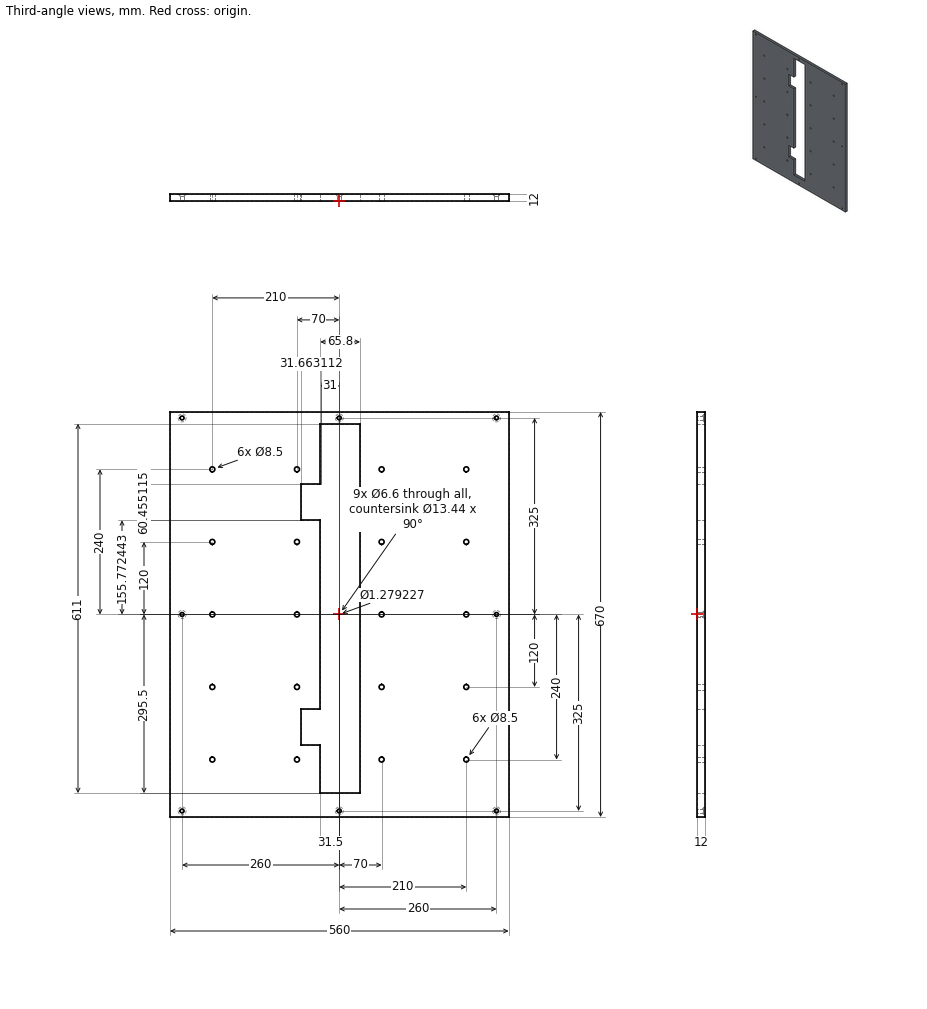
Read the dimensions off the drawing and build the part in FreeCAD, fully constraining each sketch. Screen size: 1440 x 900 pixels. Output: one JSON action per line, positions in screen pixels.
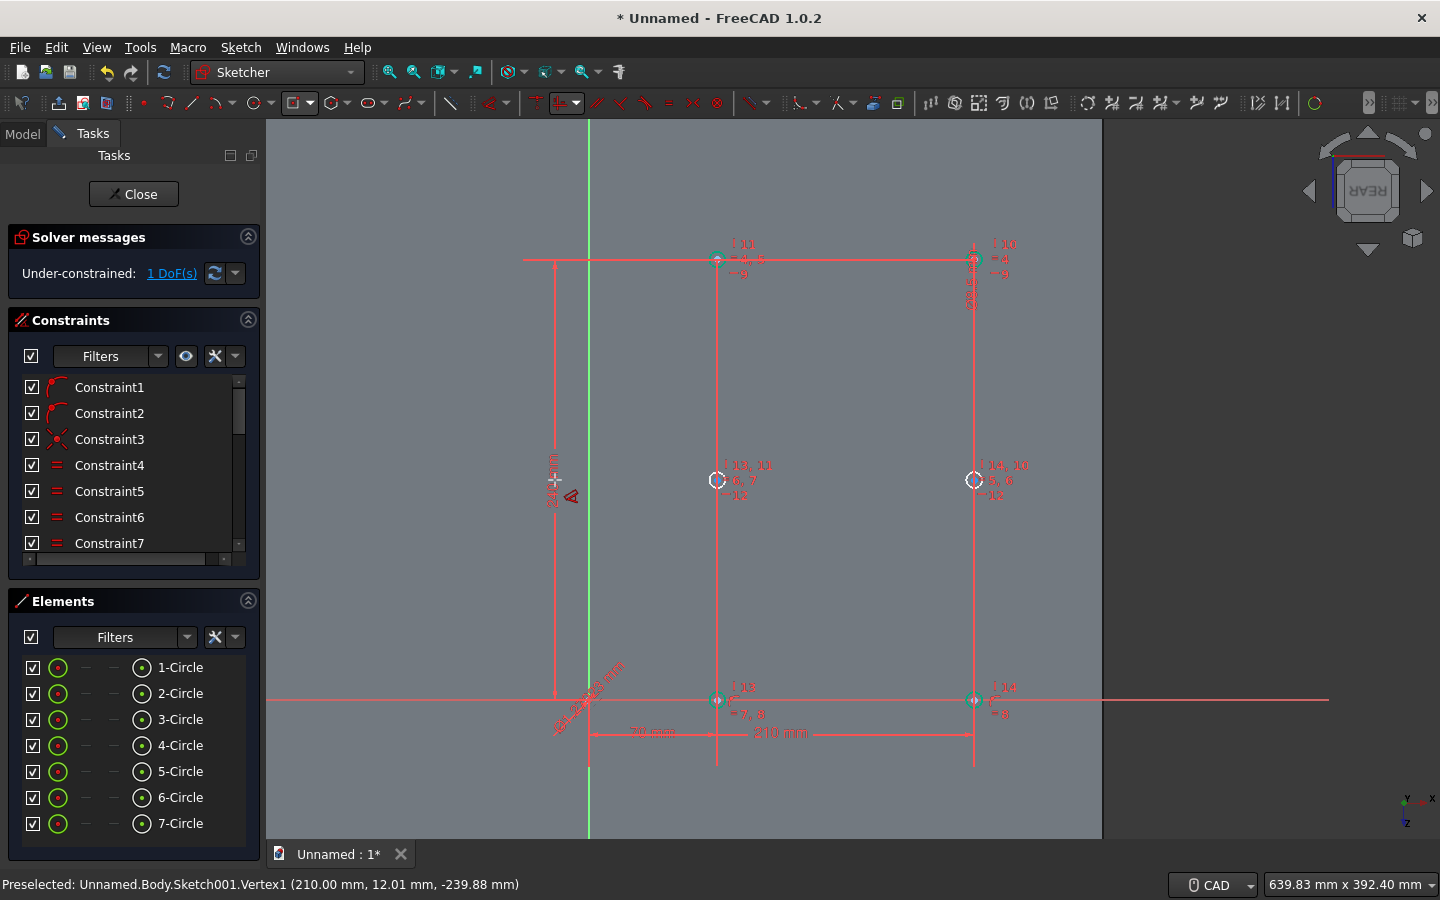
{"action": "left_click", "coordinate": [974, 480]}
{"action": "left_click", "coordinate": [555, 590]}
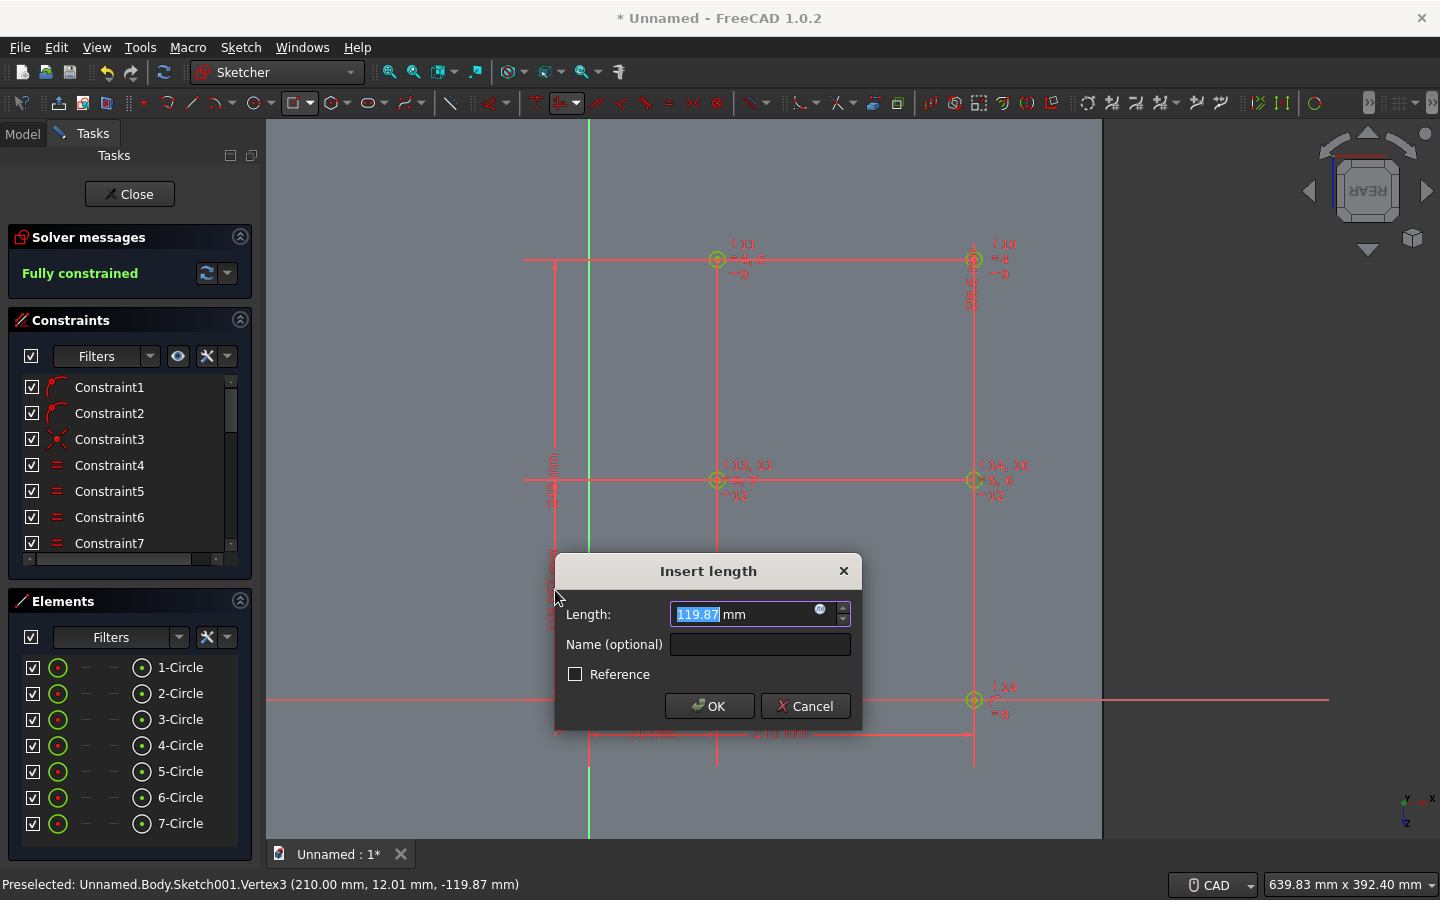
{"action": "type", "text": "120"}
{"action": "key", "text": "Return"}
{"action": "key", "text": "Escape"}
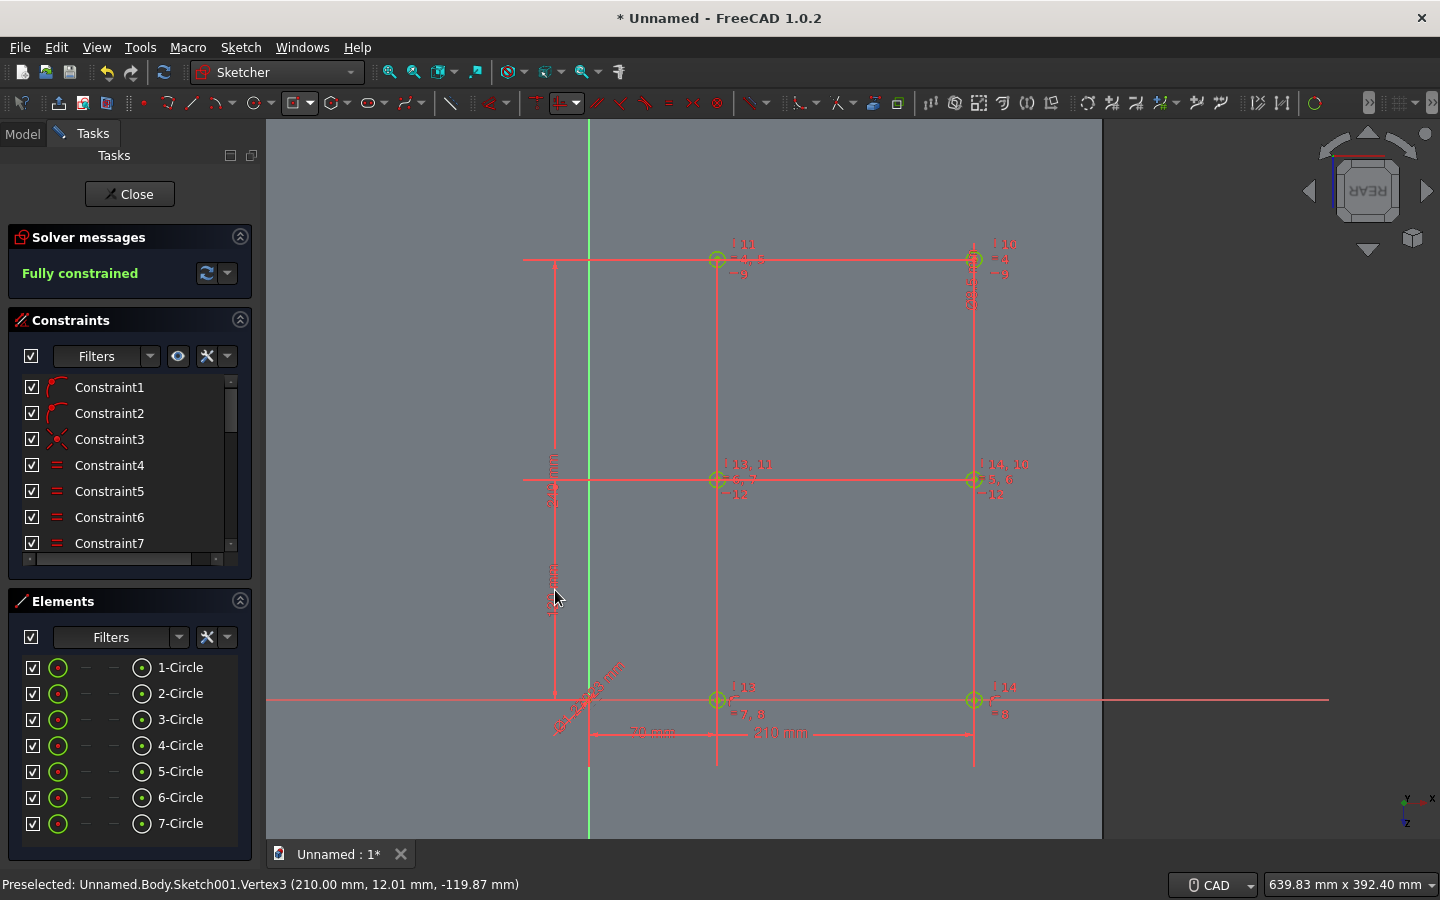
{"action": "left_click", "coordinate": [130, 194]}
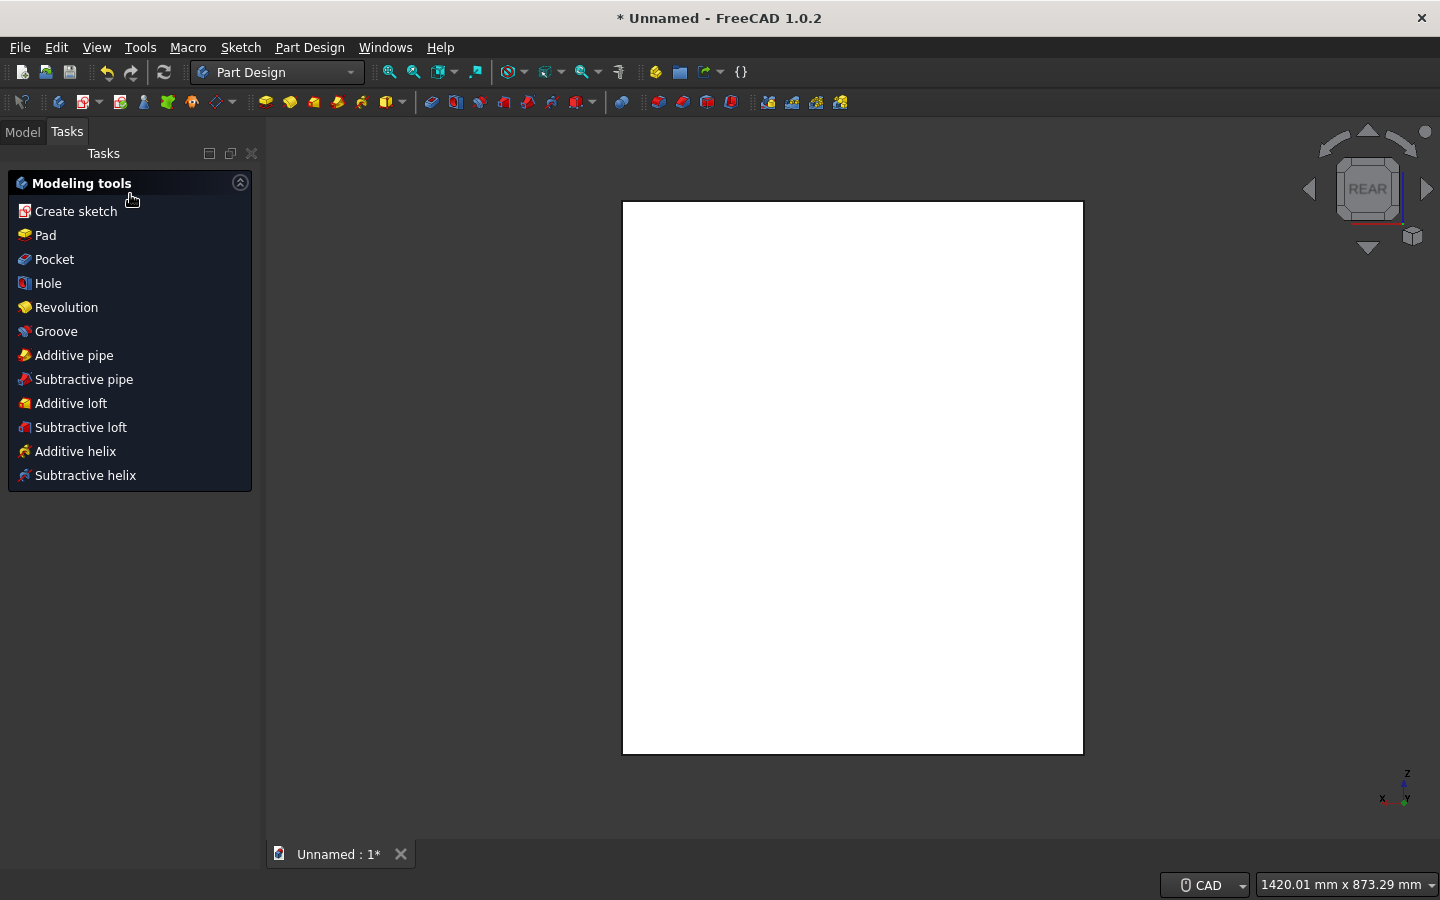
{"action": "left_click", "coordinate": [432, 102]}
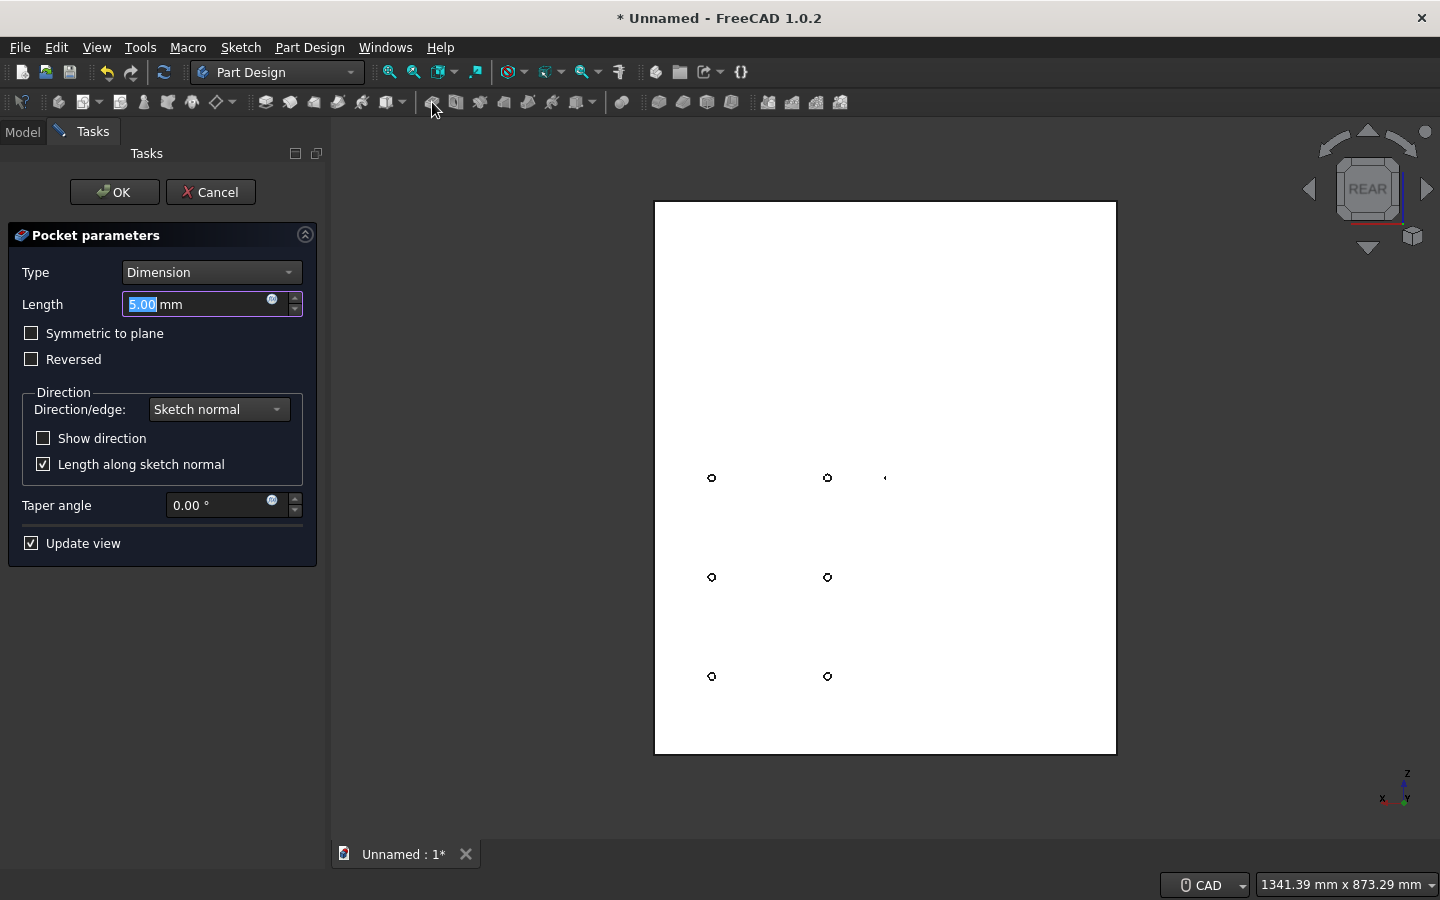
{"action": "type", "text": "12"}
{"action": "key", "text": "Tab"}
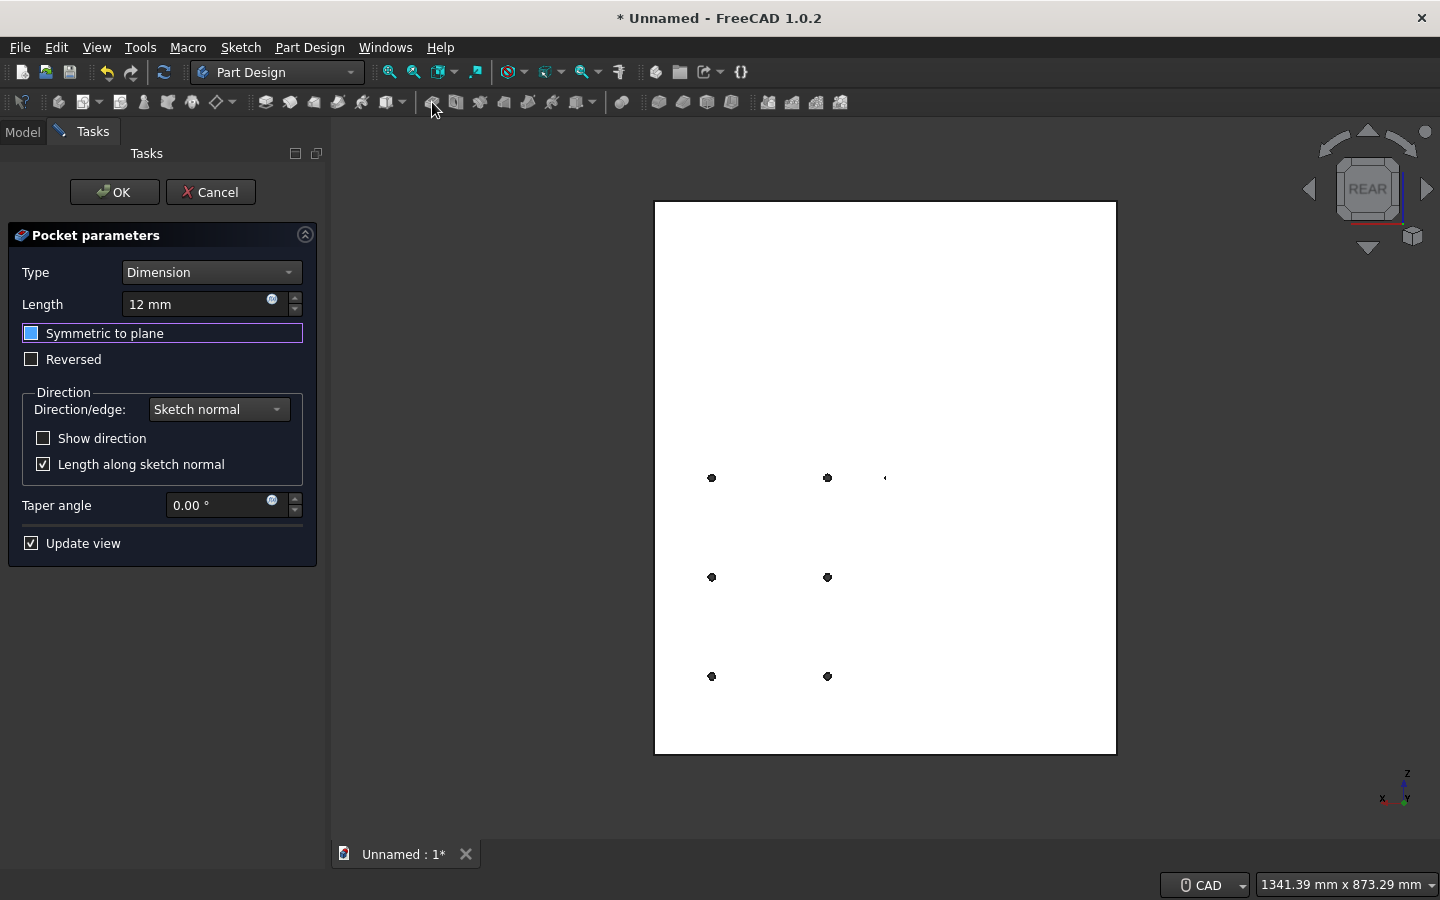
{"action": "left_click", "coordinate": [115, 192]}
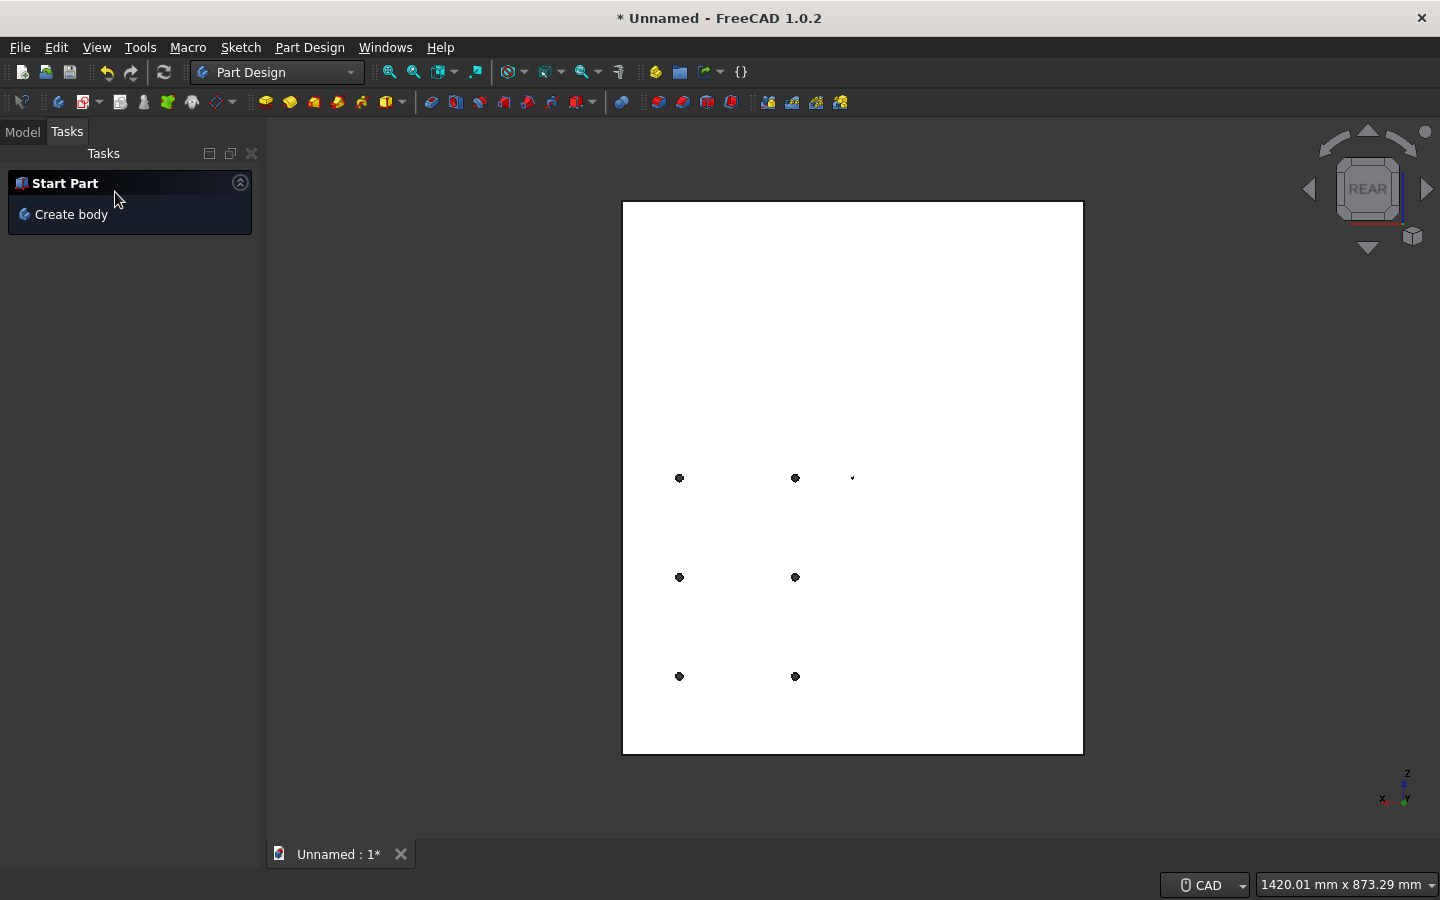
{"action": "left_click", "coordinate": [23, 131]}